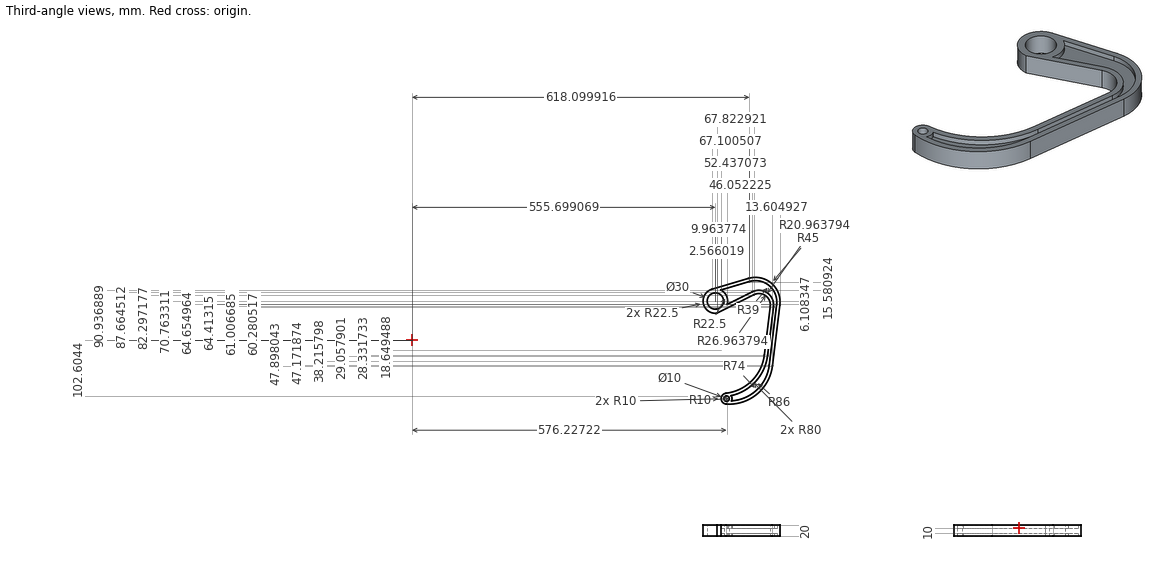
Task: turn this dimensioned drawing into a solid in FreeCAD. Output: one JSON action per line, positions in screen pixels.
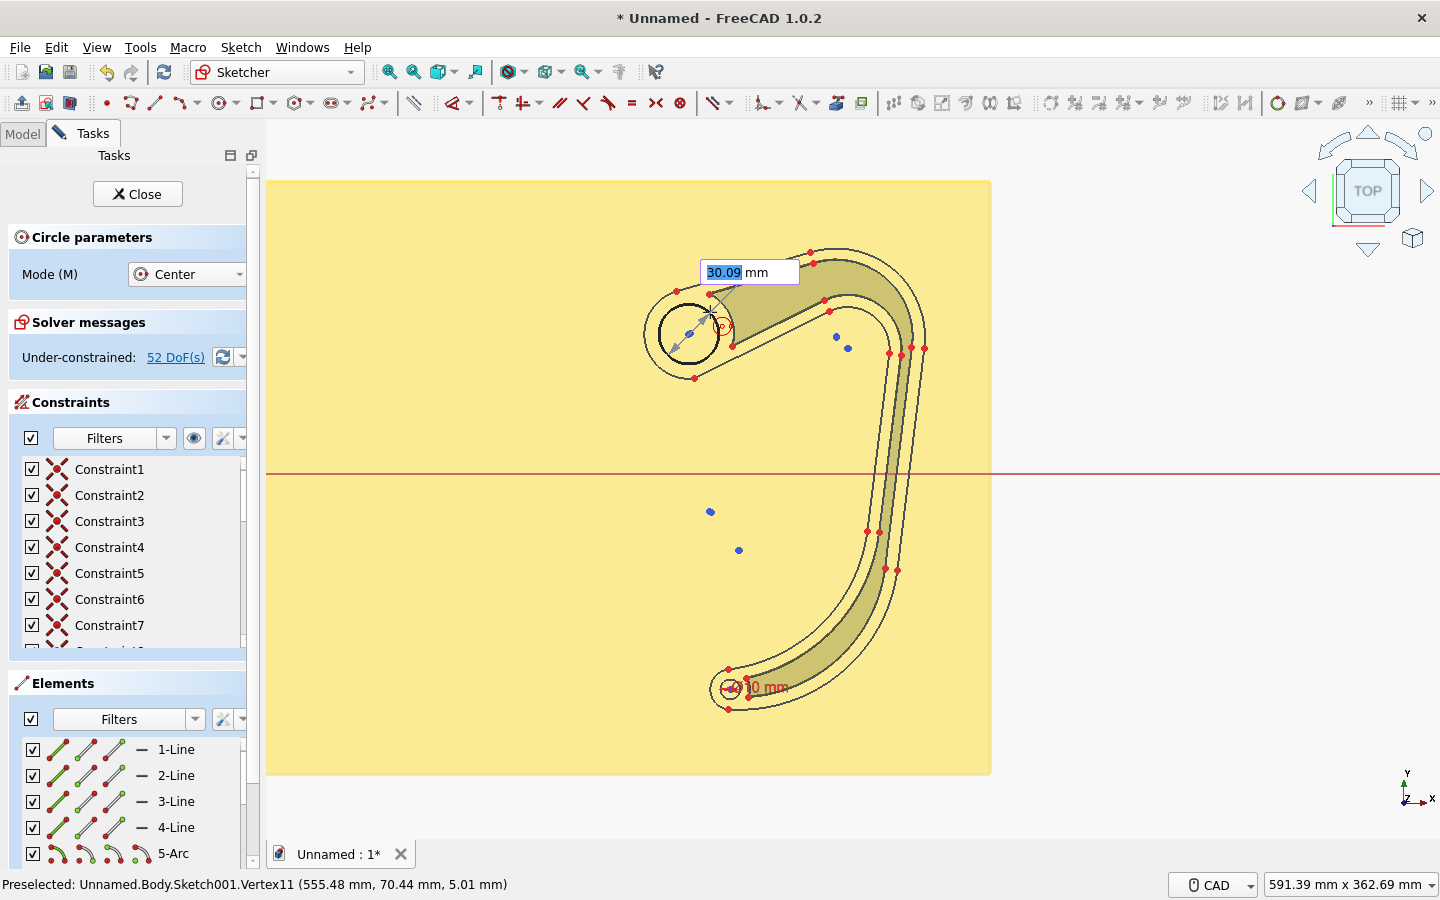
{"action": "type", "text": "30"}
{"action": "key", "text": "Return"}
{"action": "key", "text": "Escape"}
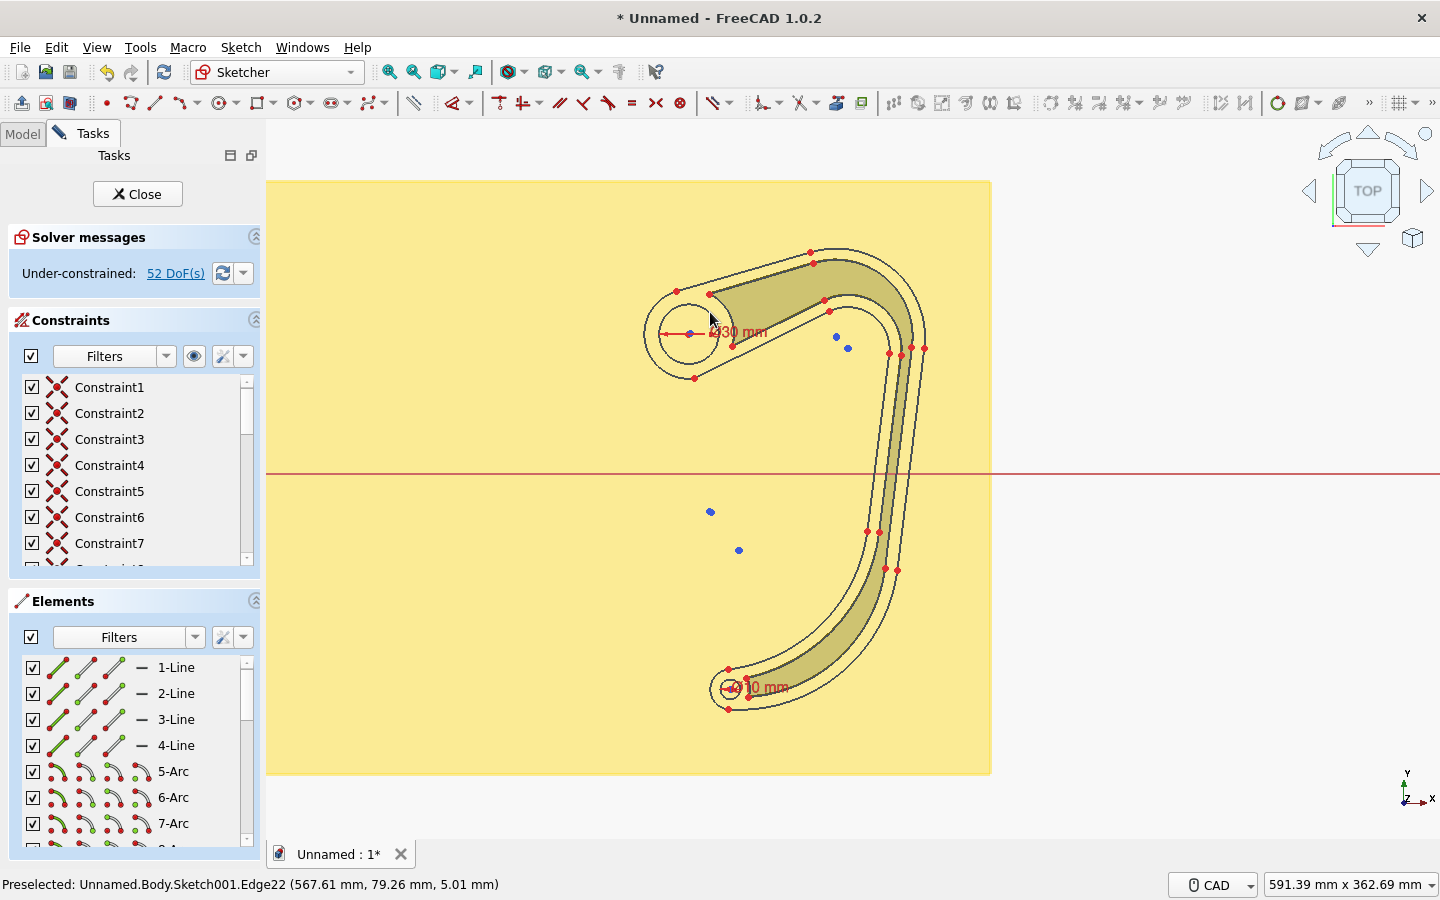
{"action": "left_click", "coordinate": [770, 264]}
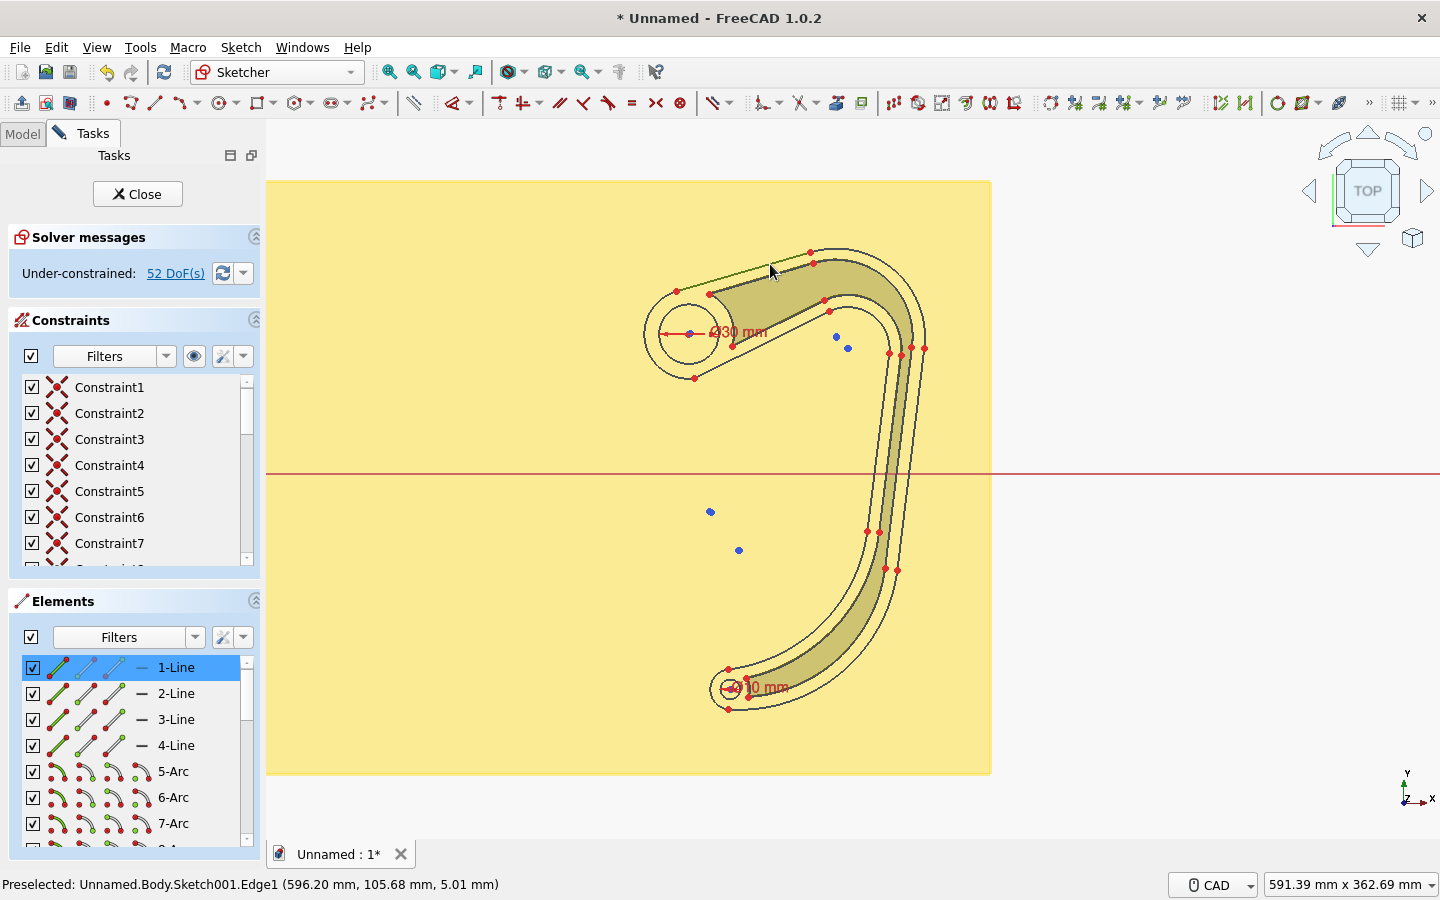
{"action": "left_click", "coordinate": [648, 317]}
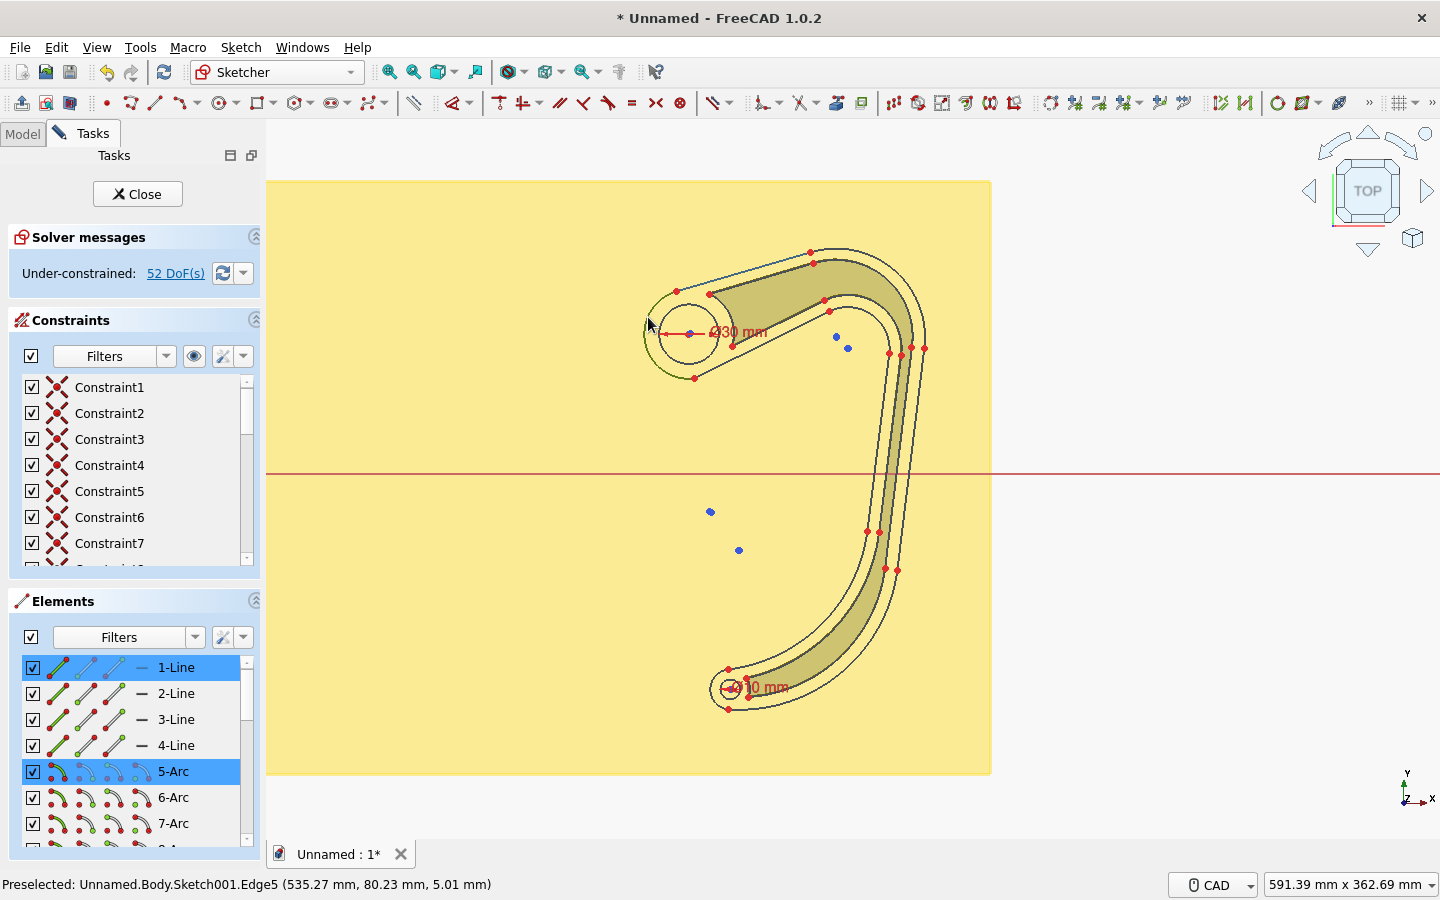
{"action": "left_click", "coordinate": [608, 104]}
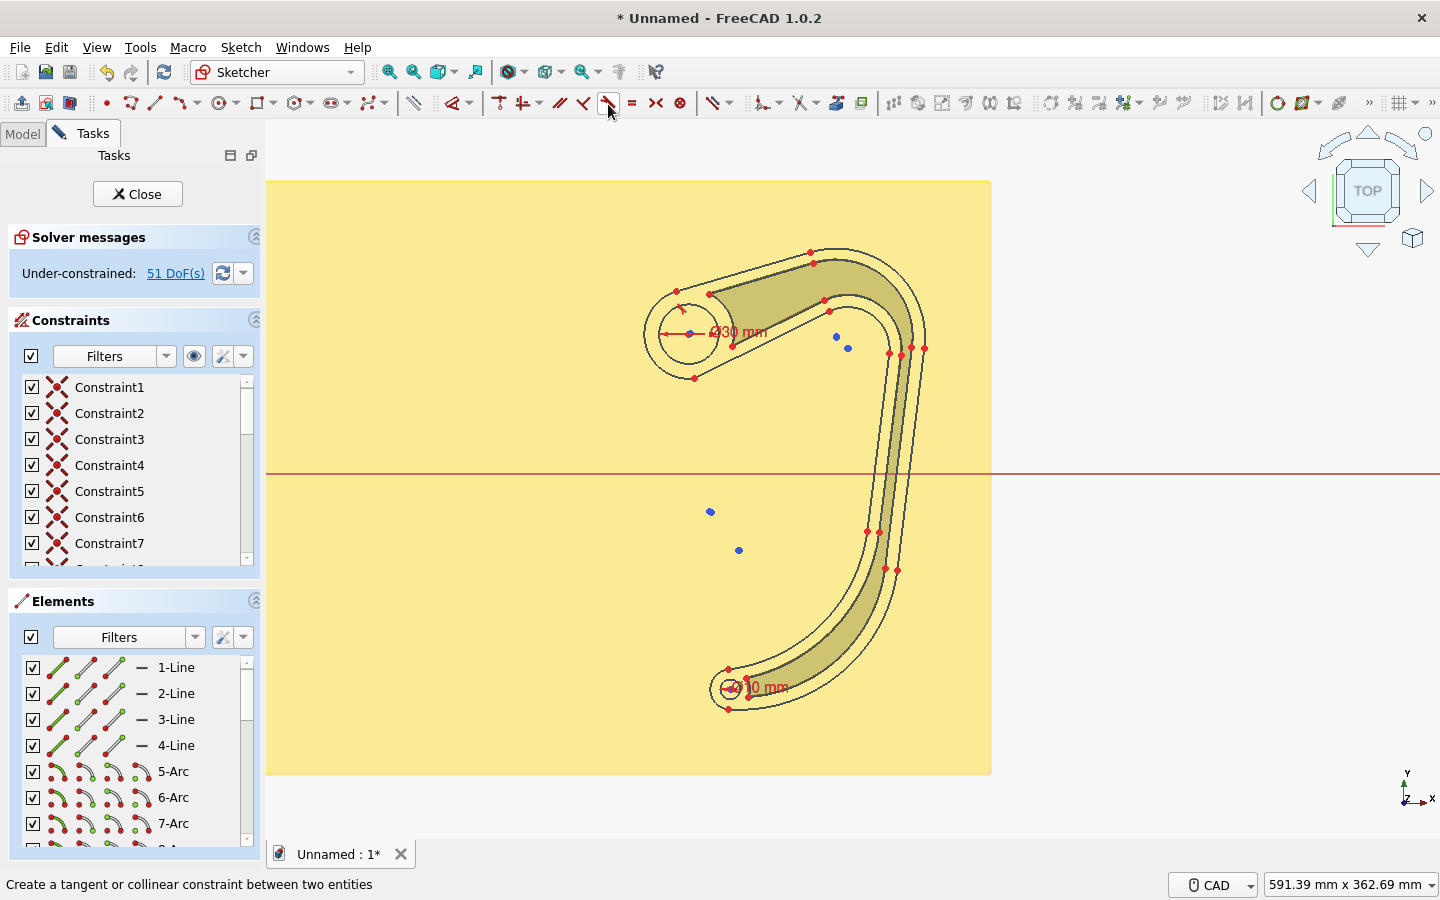
{"action": "left_click", "coordinate": [770, 264]}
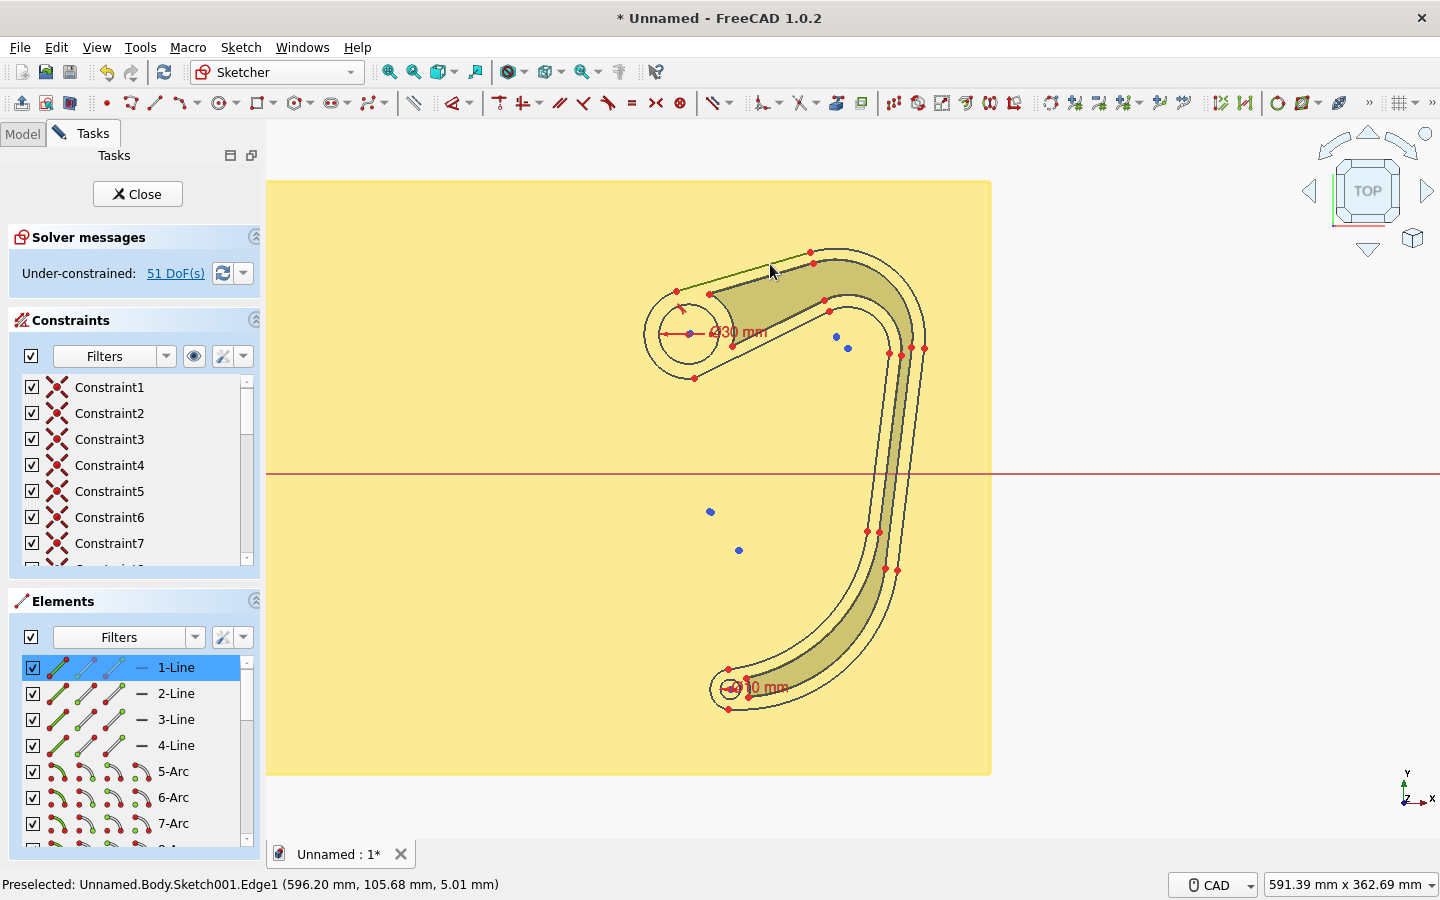
{"action": "left_click", "coordinate": [915, 297]}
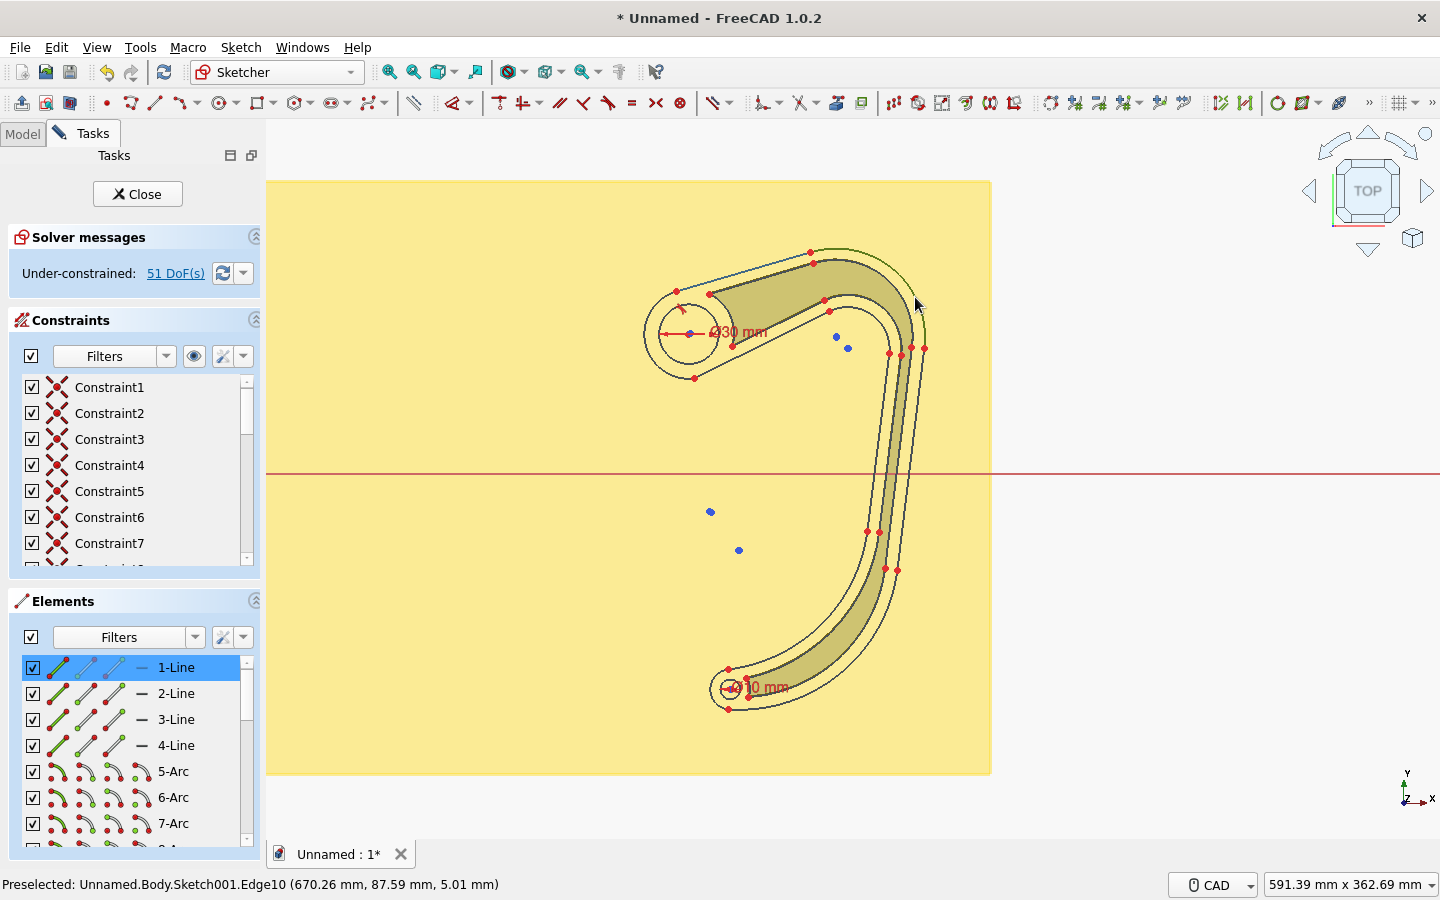
{"action": "left_click", "coordinate": [608, 104]}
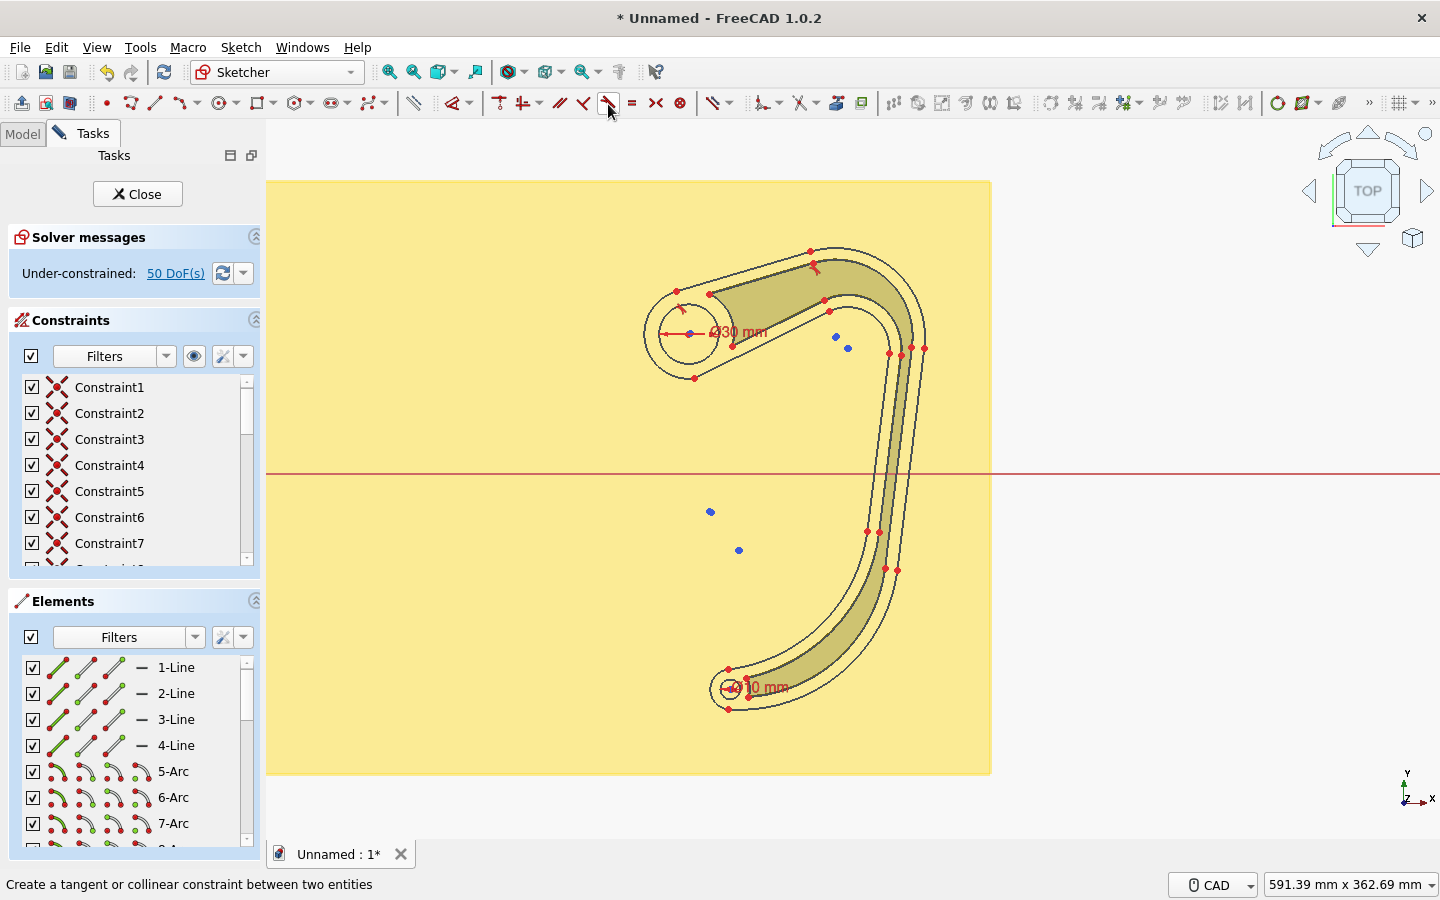
{"action": "left_click", "coordinate": [735, 358]}